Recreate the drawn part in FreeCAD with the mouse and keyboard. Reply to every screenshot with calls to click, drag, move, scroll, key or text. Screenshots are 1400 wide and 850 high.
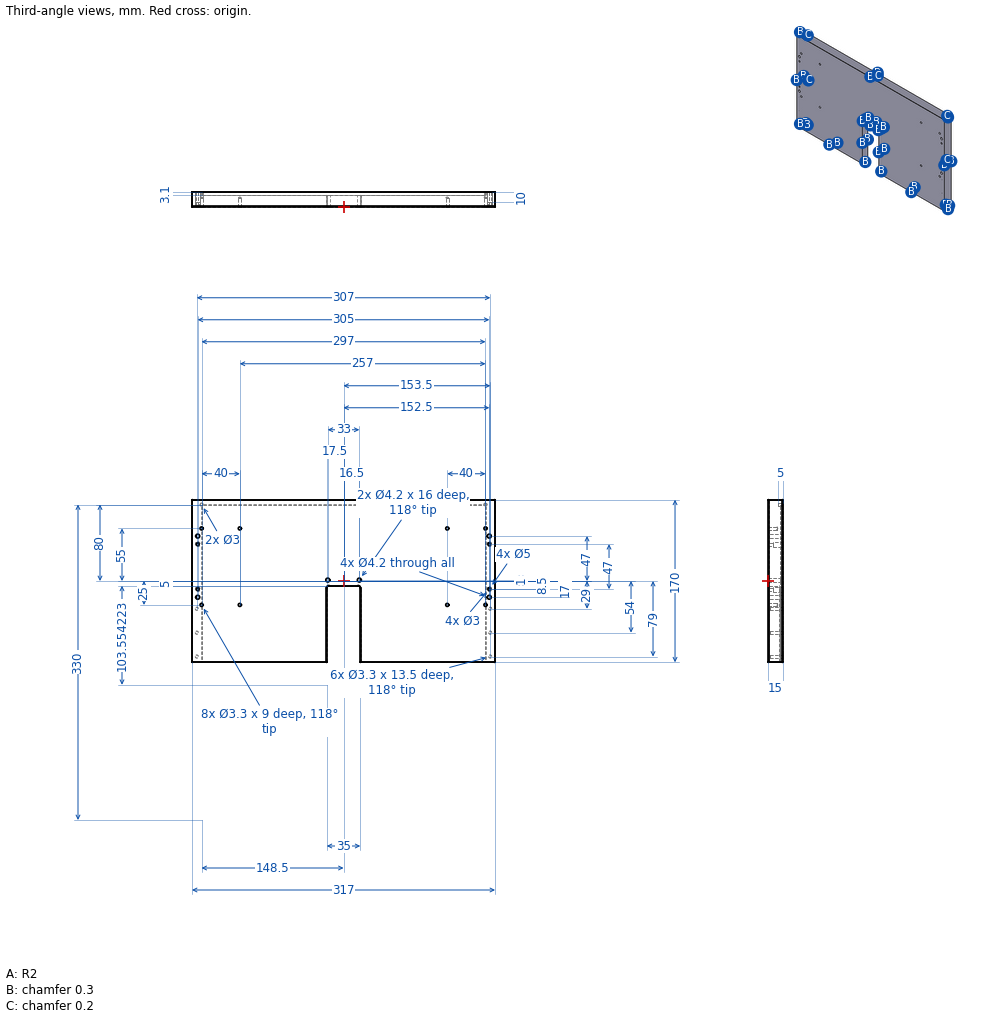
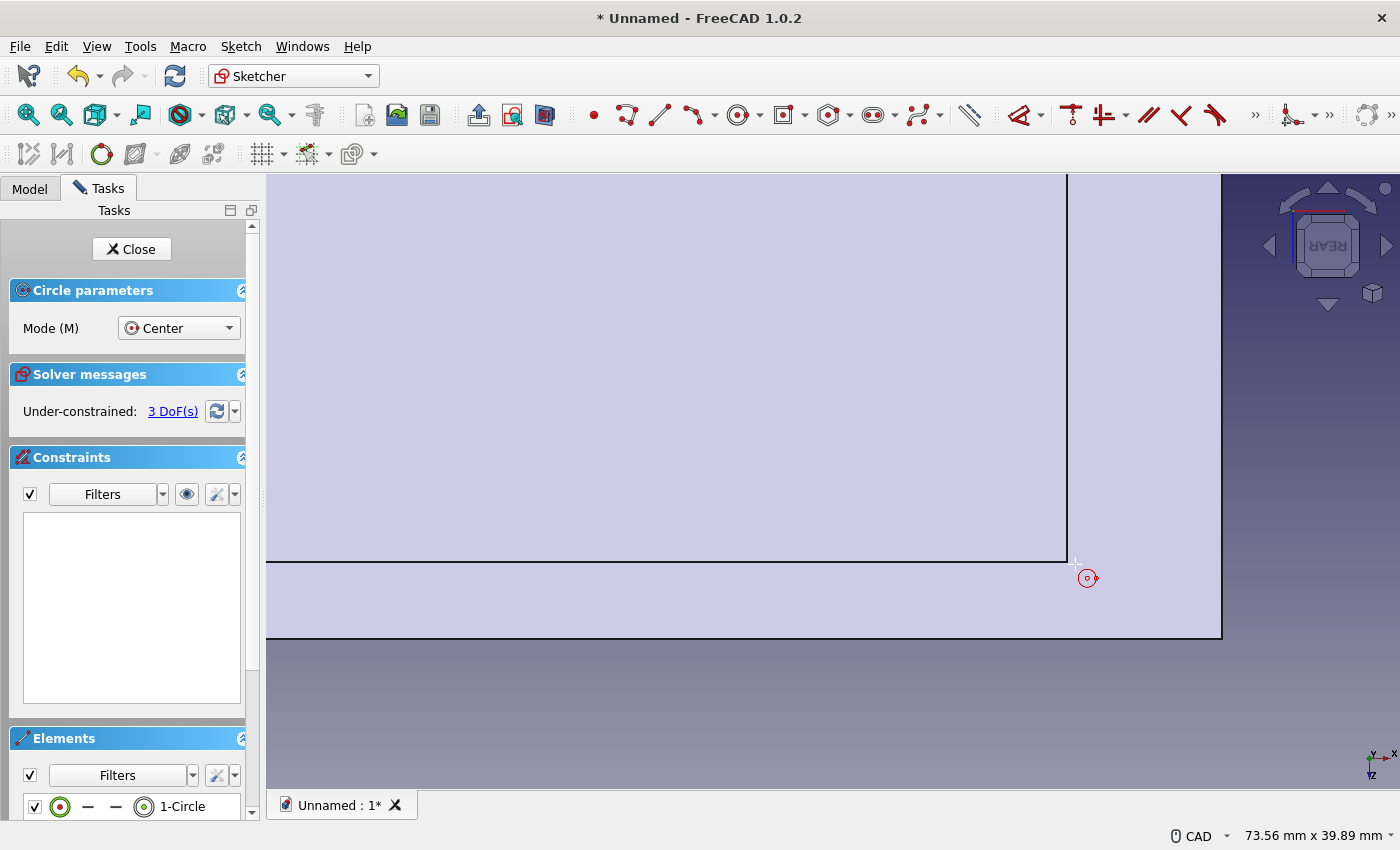
scroll(1075, 564, down, 10)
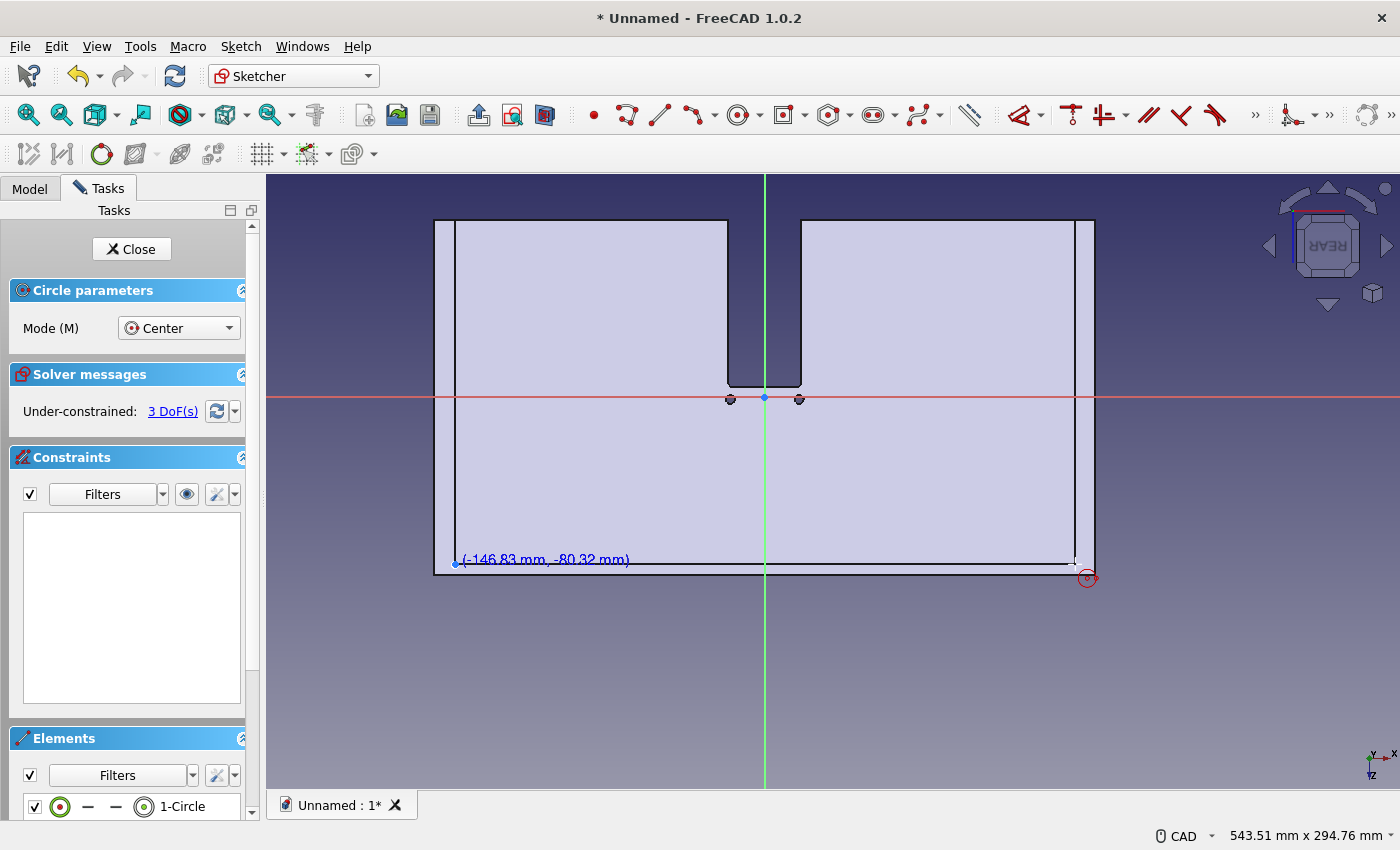
click(1075, 564)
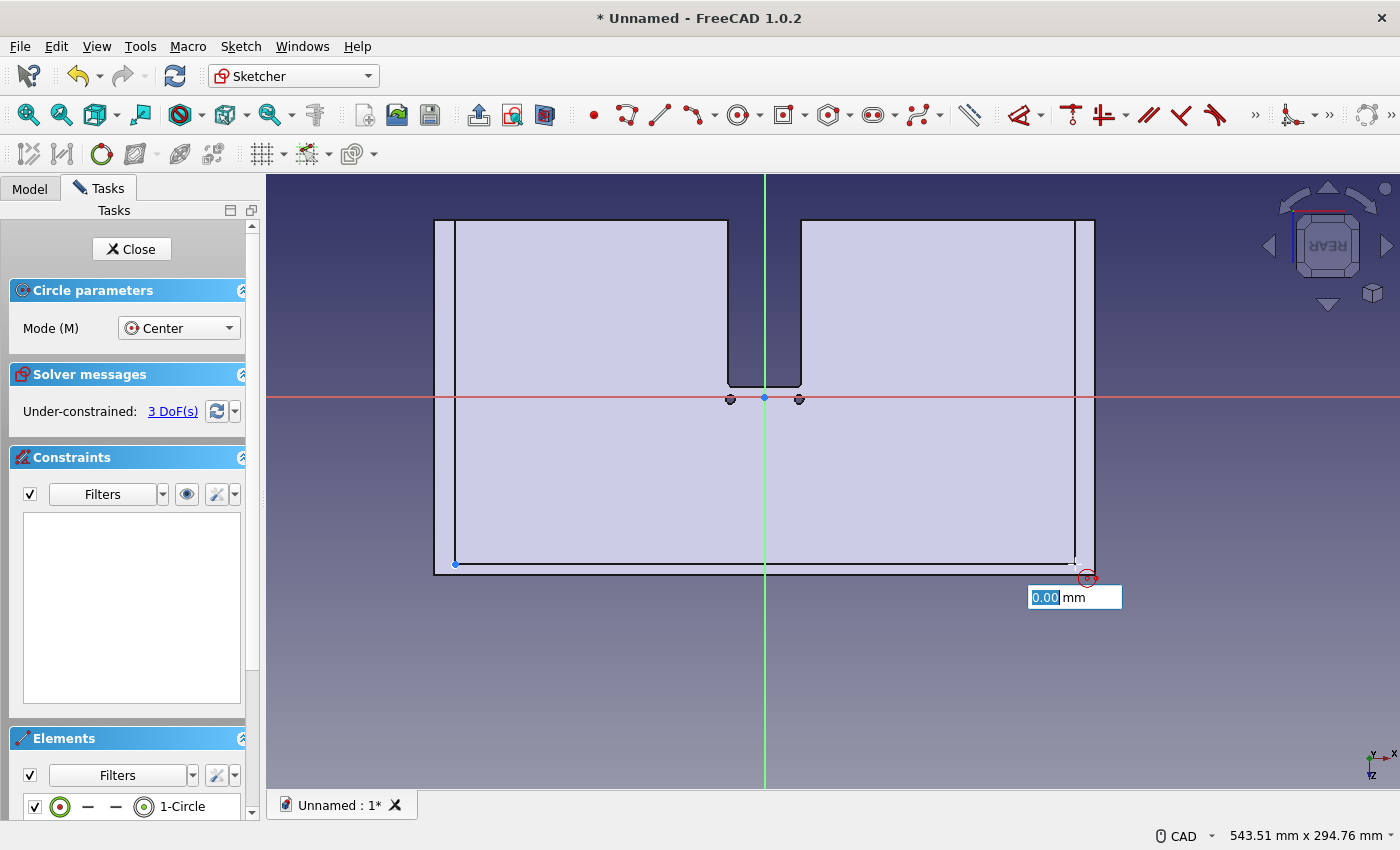
scroll(1077, 562, up, 9)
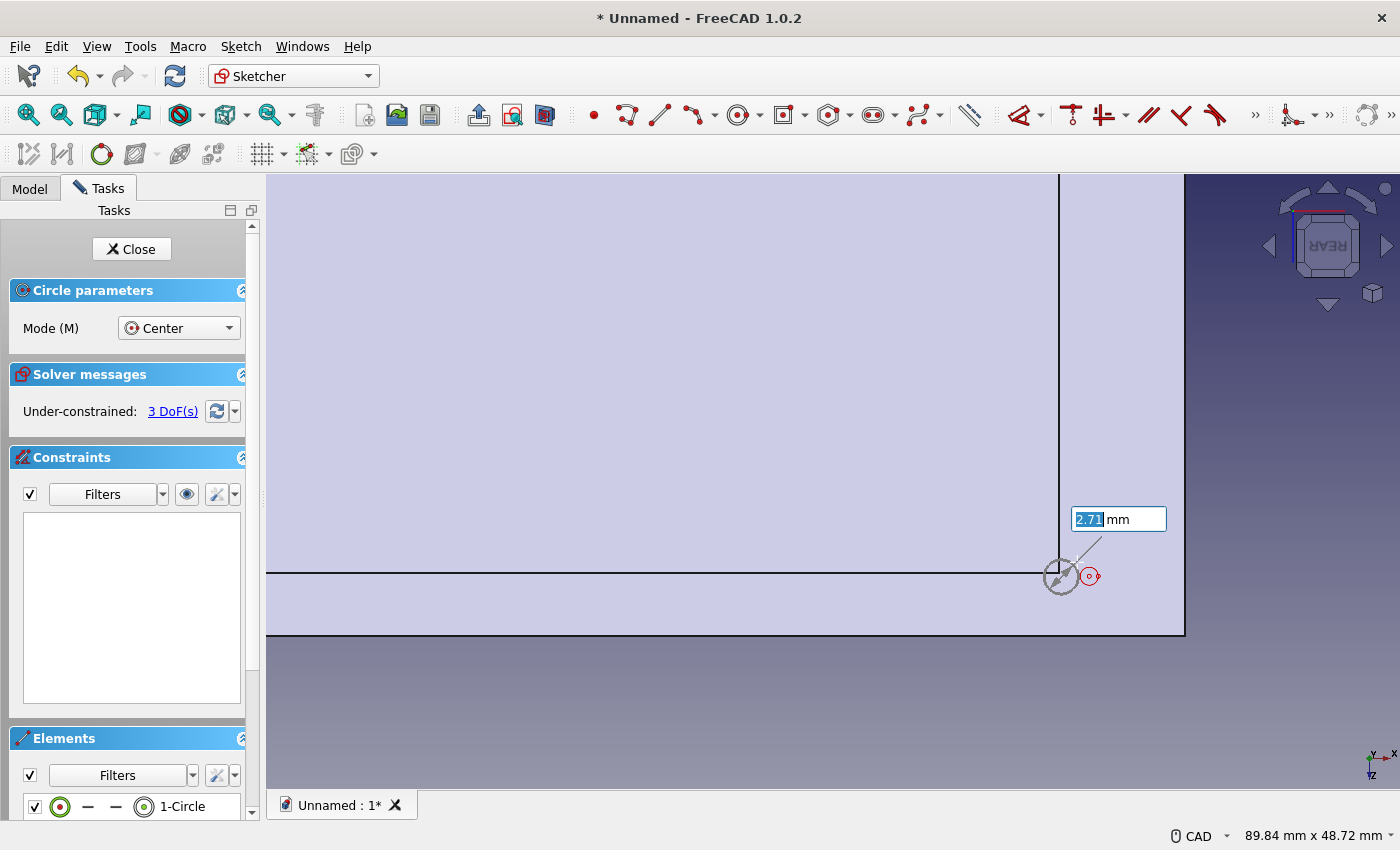
click(1072, 560)
key(Escape)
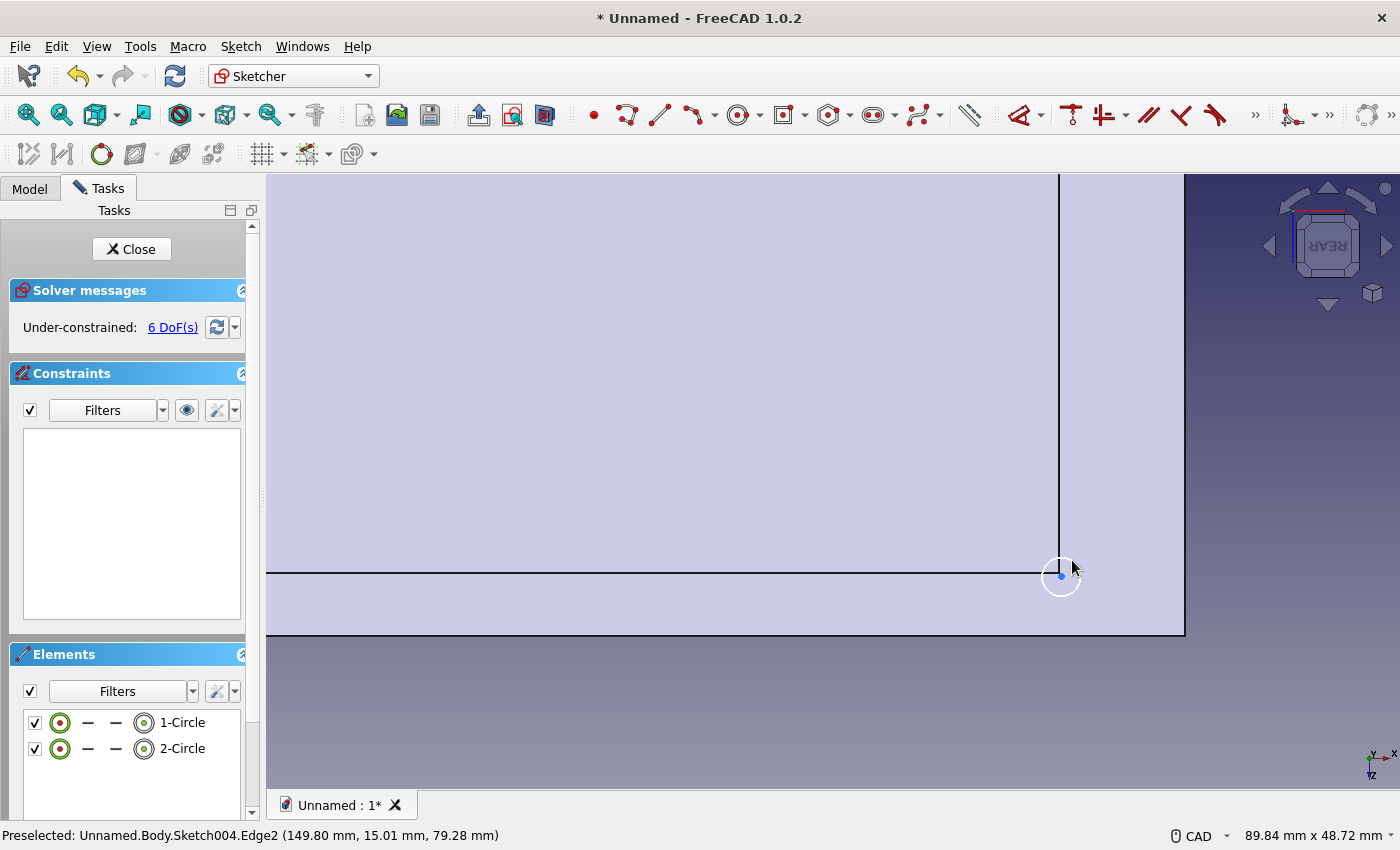
scroll(1077, 562, down, 9)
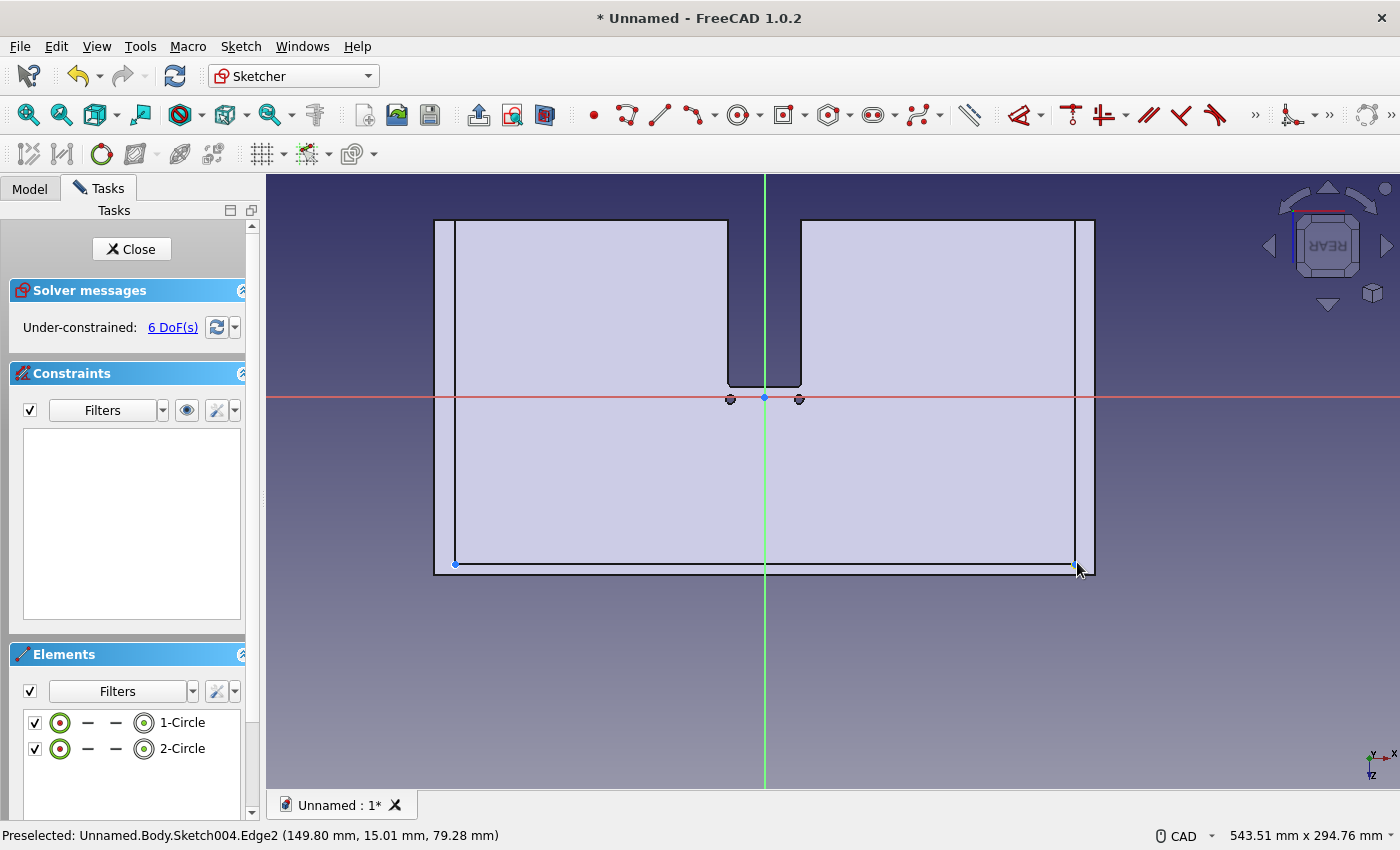
scroll(457, 563, up, 8)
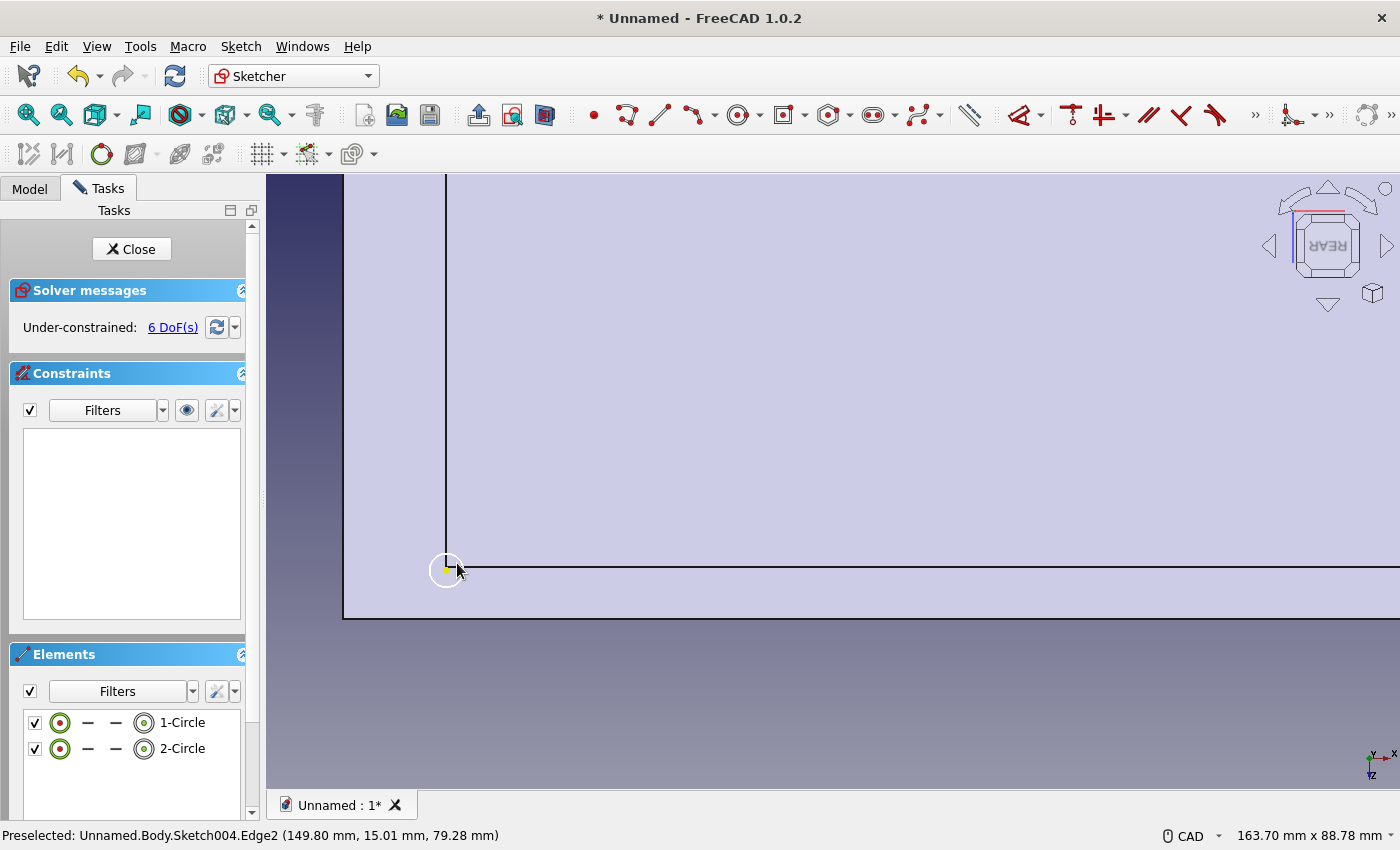
click(458, 558)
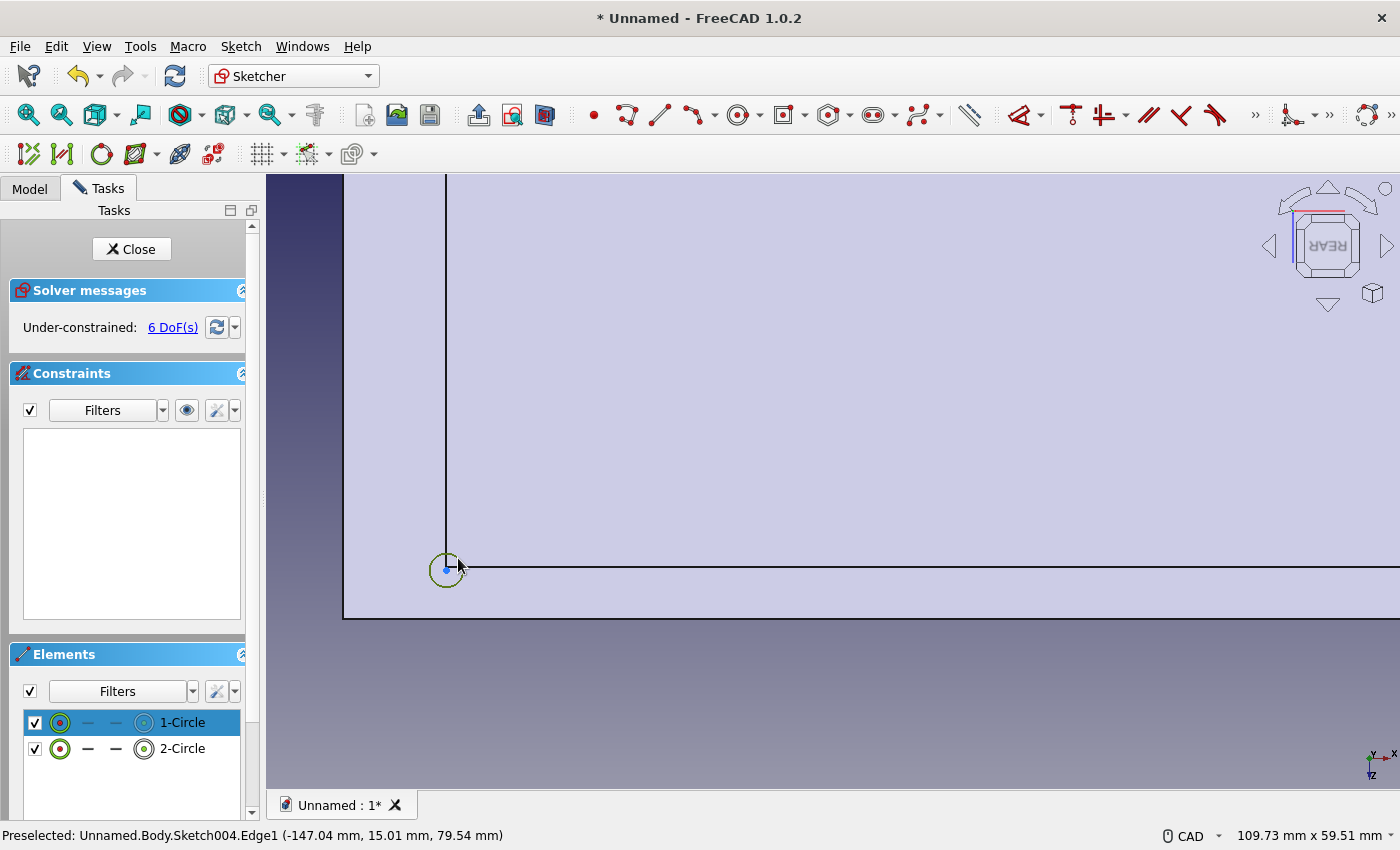
scroll(457, 562, down, 8)